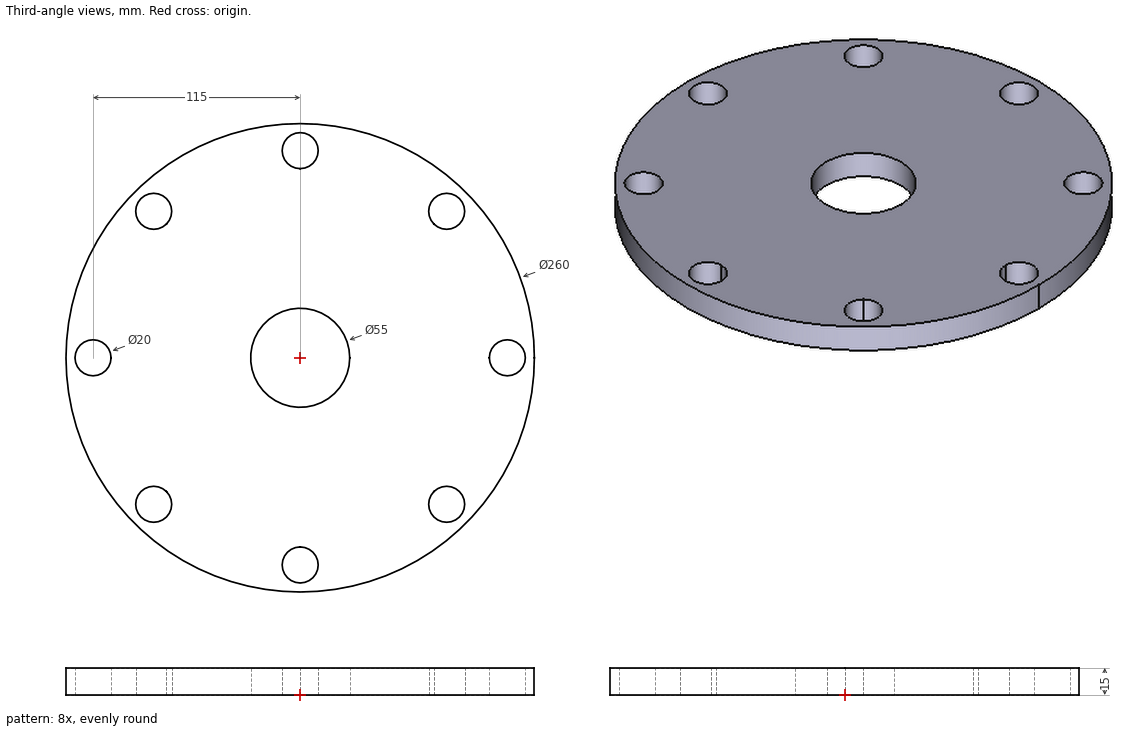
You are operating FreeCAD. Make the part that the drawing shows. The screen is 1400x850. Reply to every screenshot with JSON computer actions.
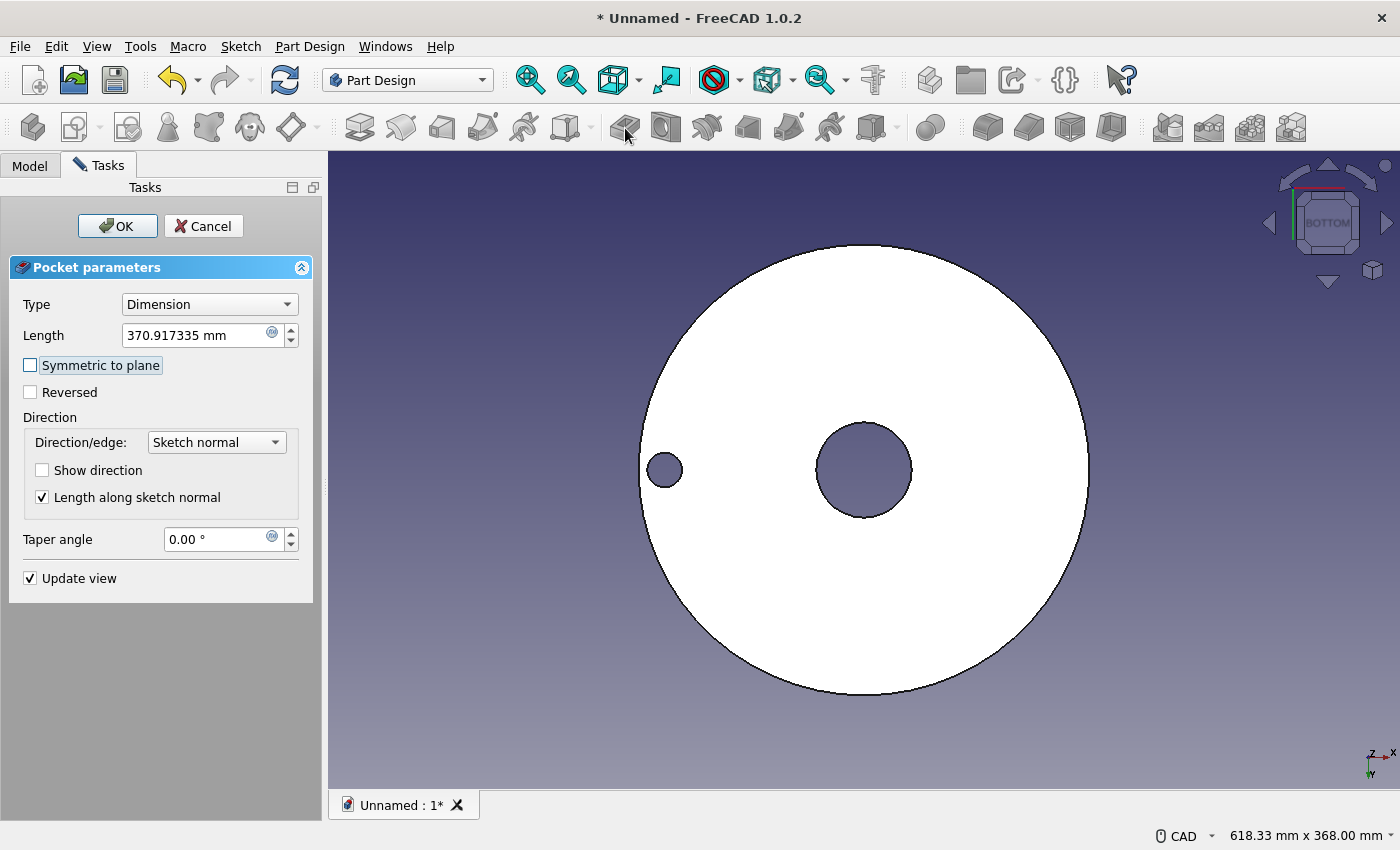
{"action": "left_click", "coordinate": [31, 365]}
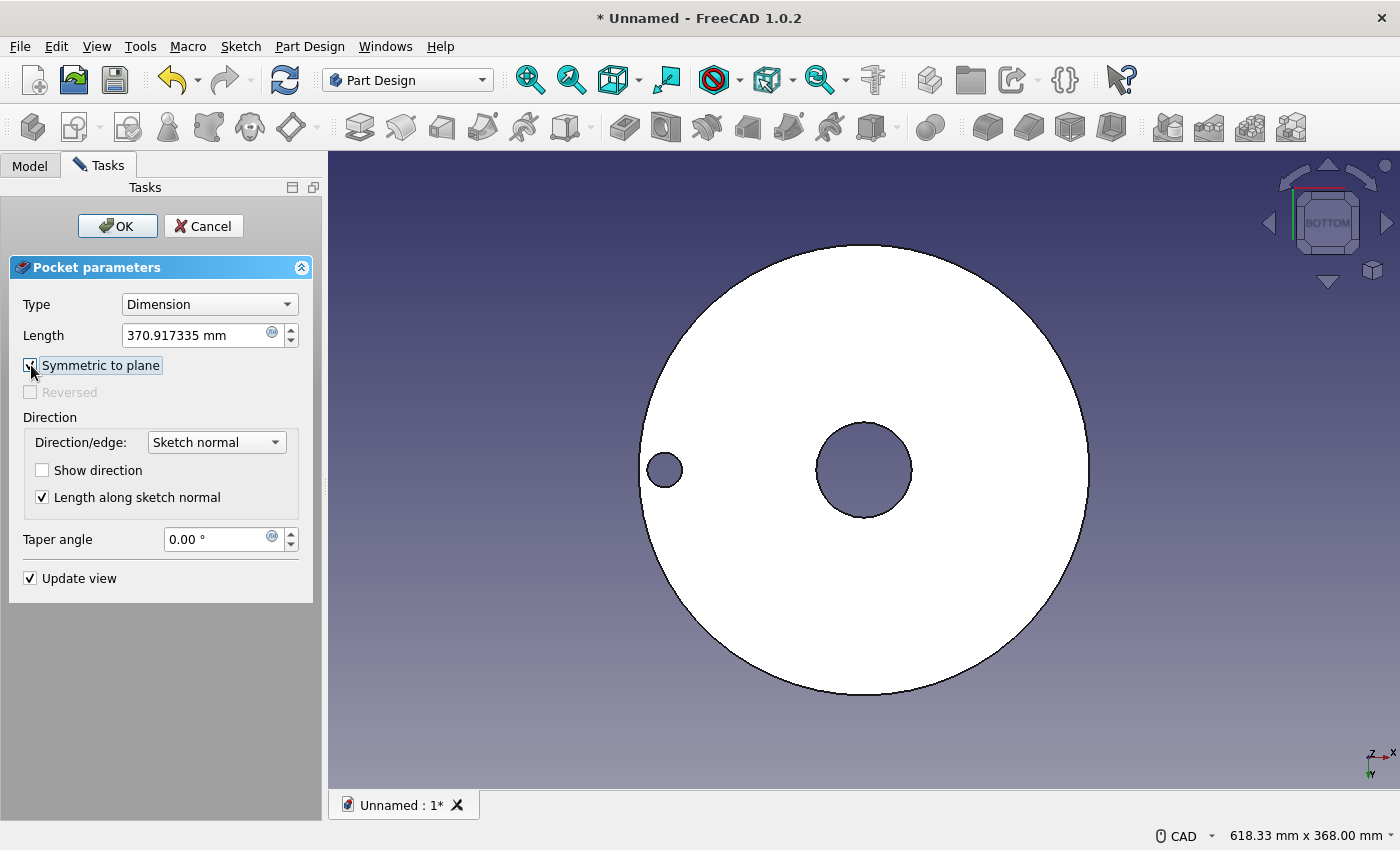
{"action": "left_click", "coordinate": [118, 226]}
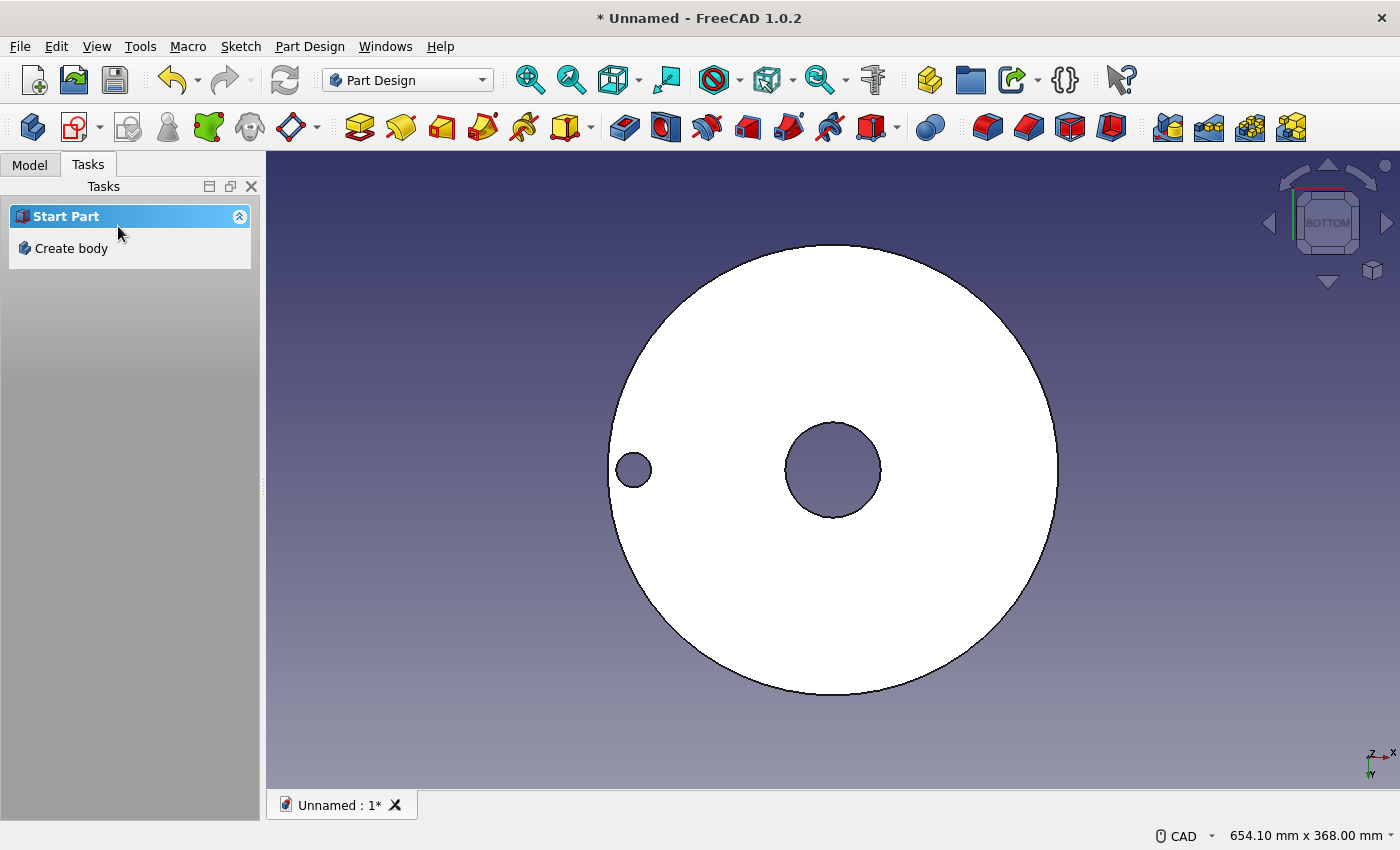
{"action": "left_click", "coordinate": [30, 164]}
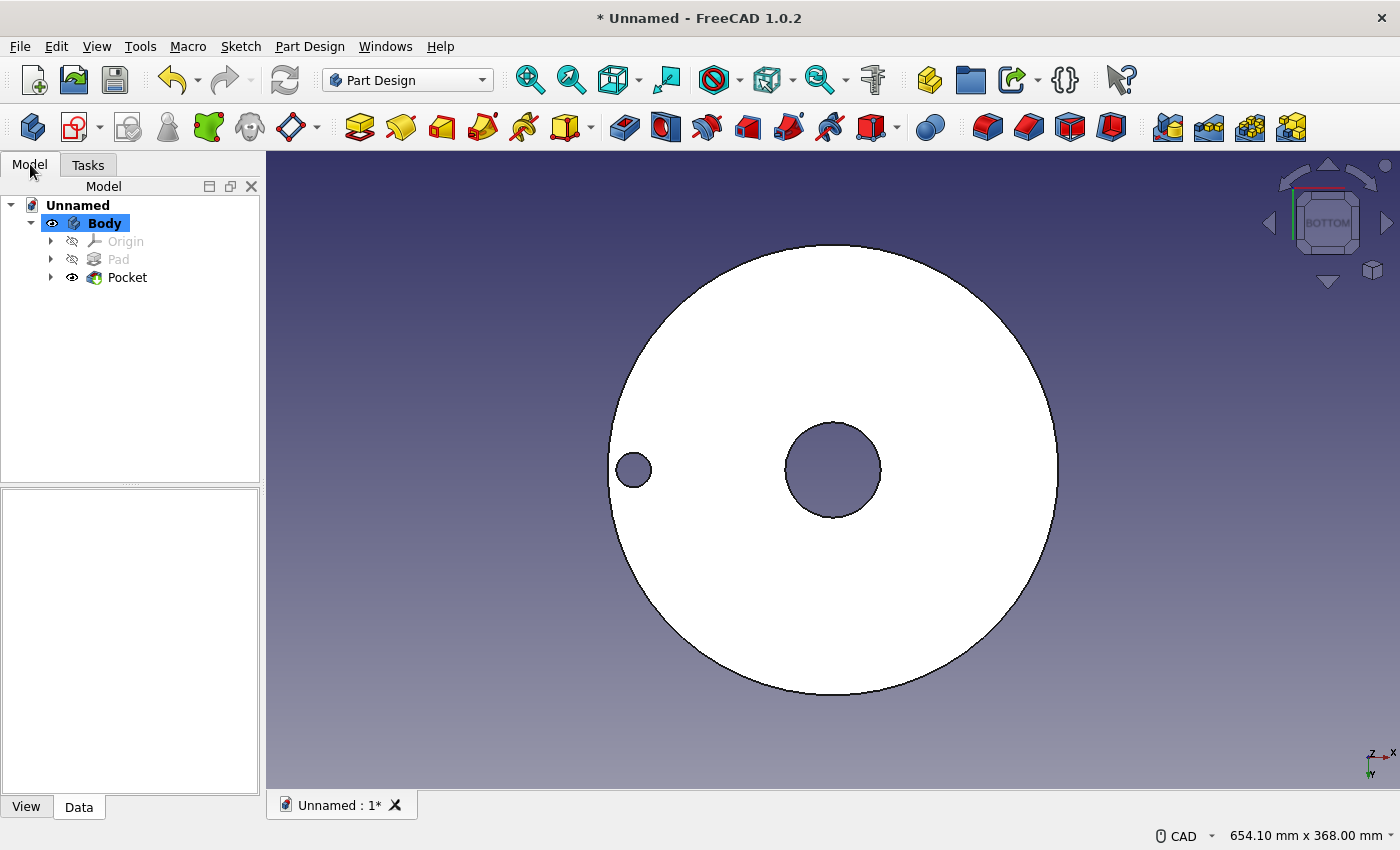
{"action": "left_click", "coordinate": [117, 277]}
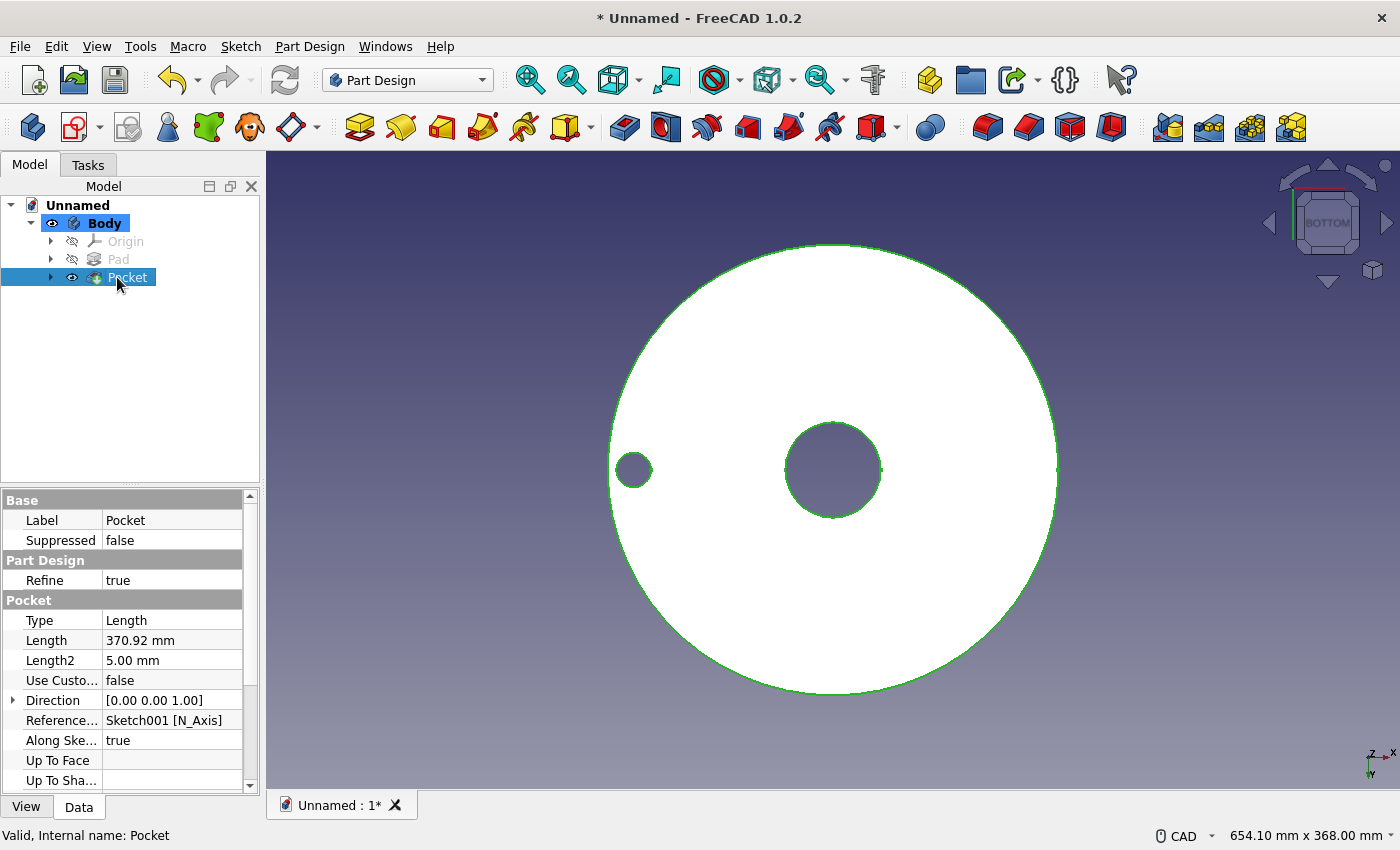
{"action": "left_click", "coordinate": [1250, 128]}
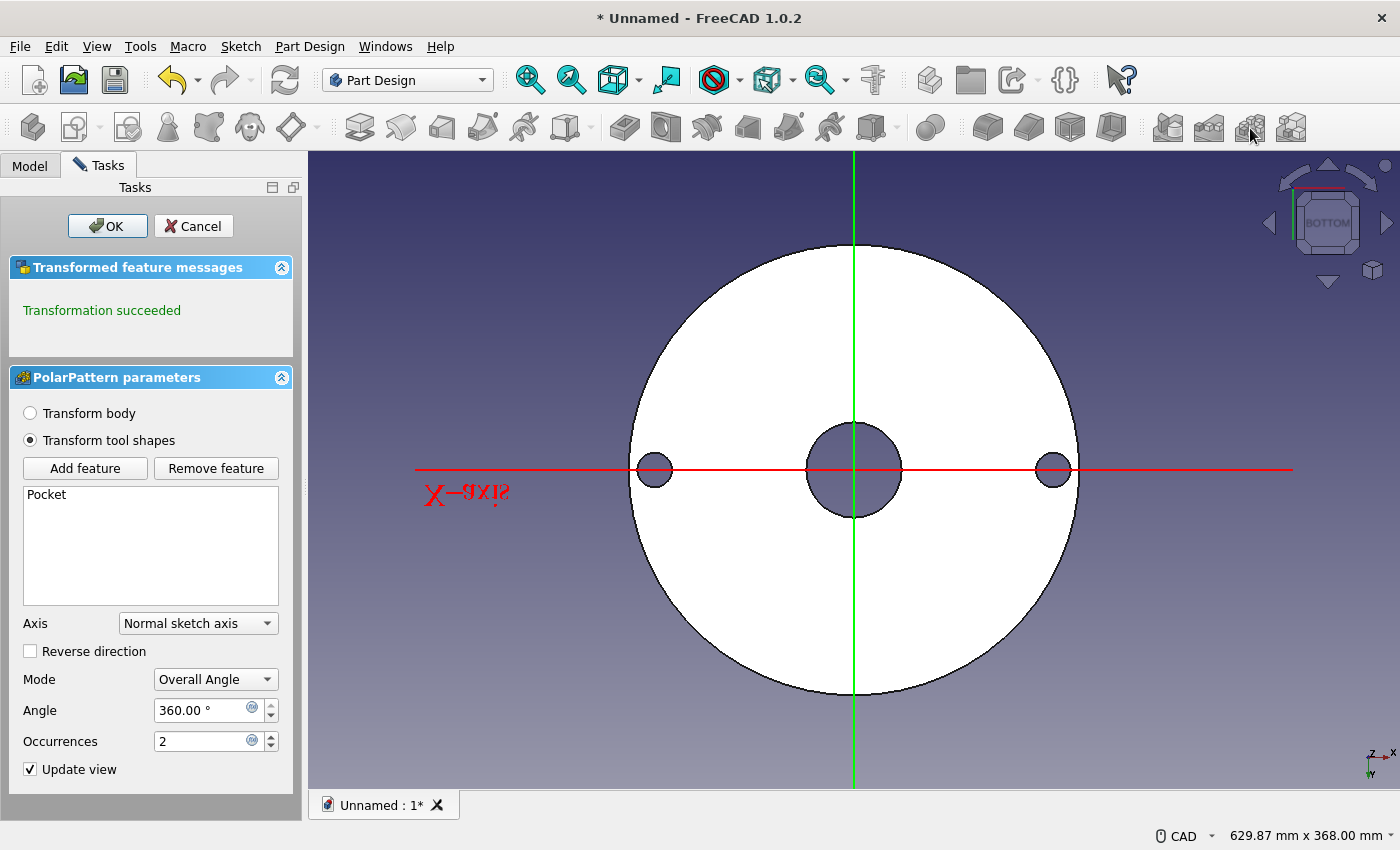
{"action": "left_click", "coordinate": [199, 624]}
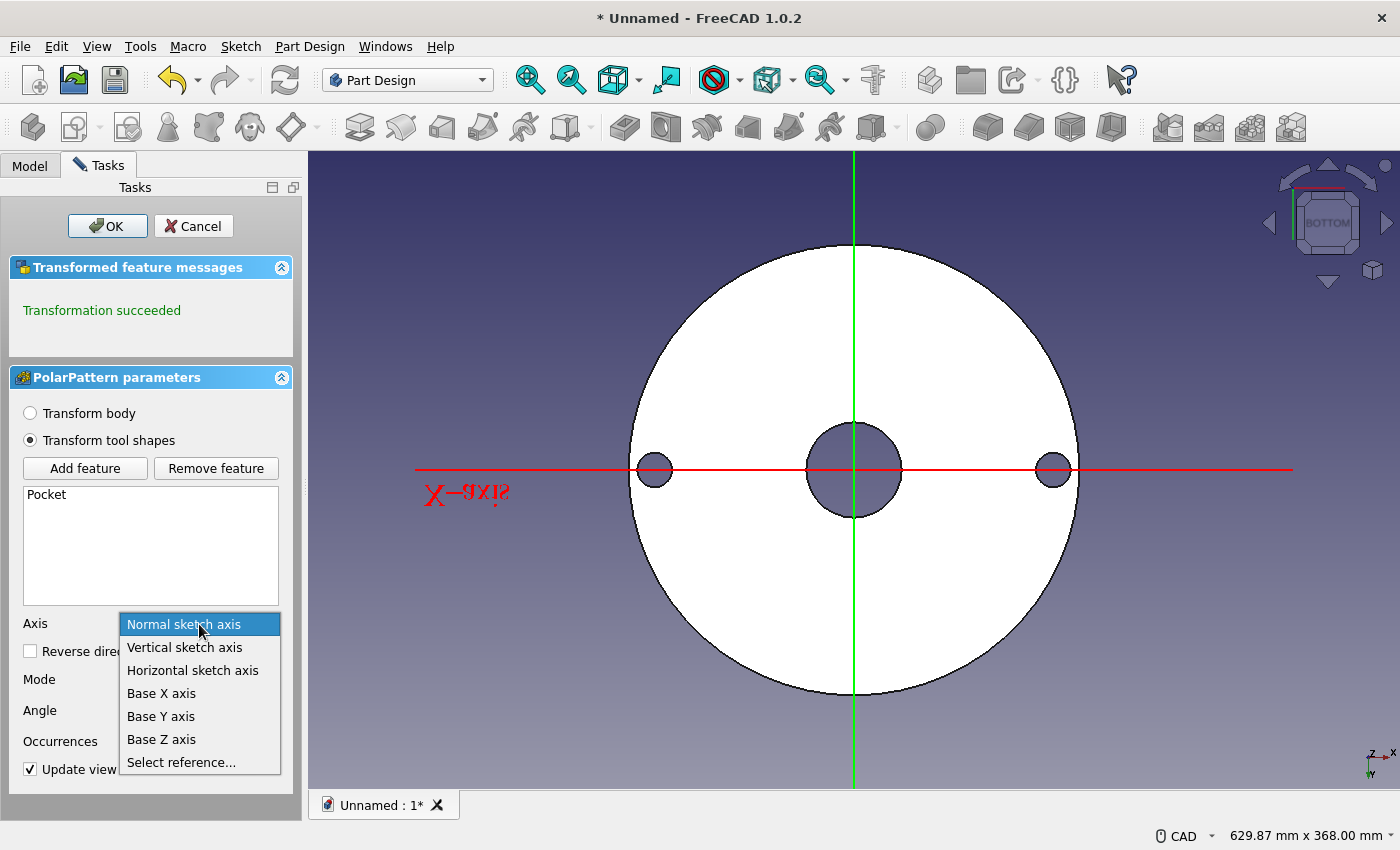
{"action": "left_click", "coordinate": [198, 740]}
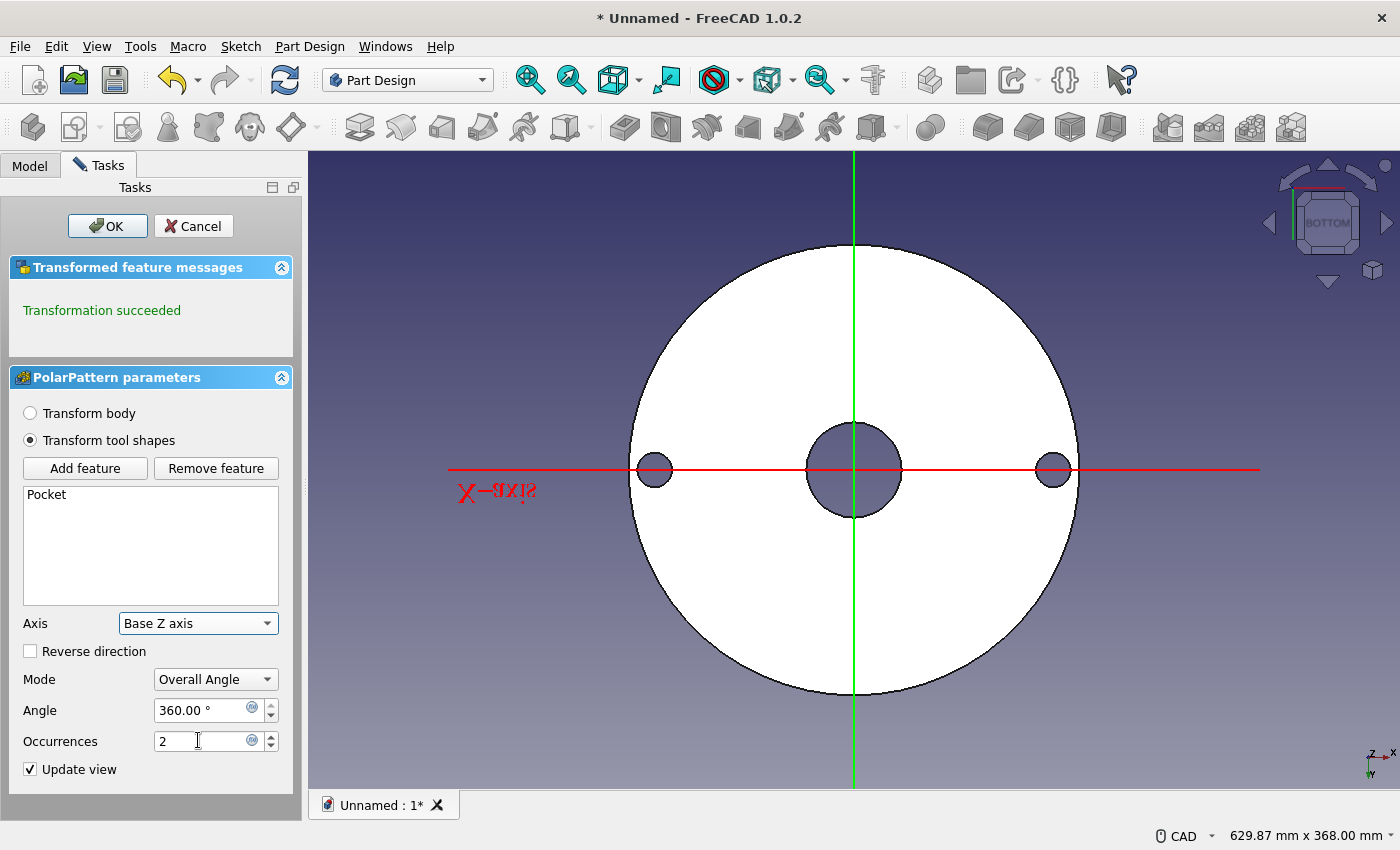
{"action": "triple_click", "coordinate": [210, 742]}